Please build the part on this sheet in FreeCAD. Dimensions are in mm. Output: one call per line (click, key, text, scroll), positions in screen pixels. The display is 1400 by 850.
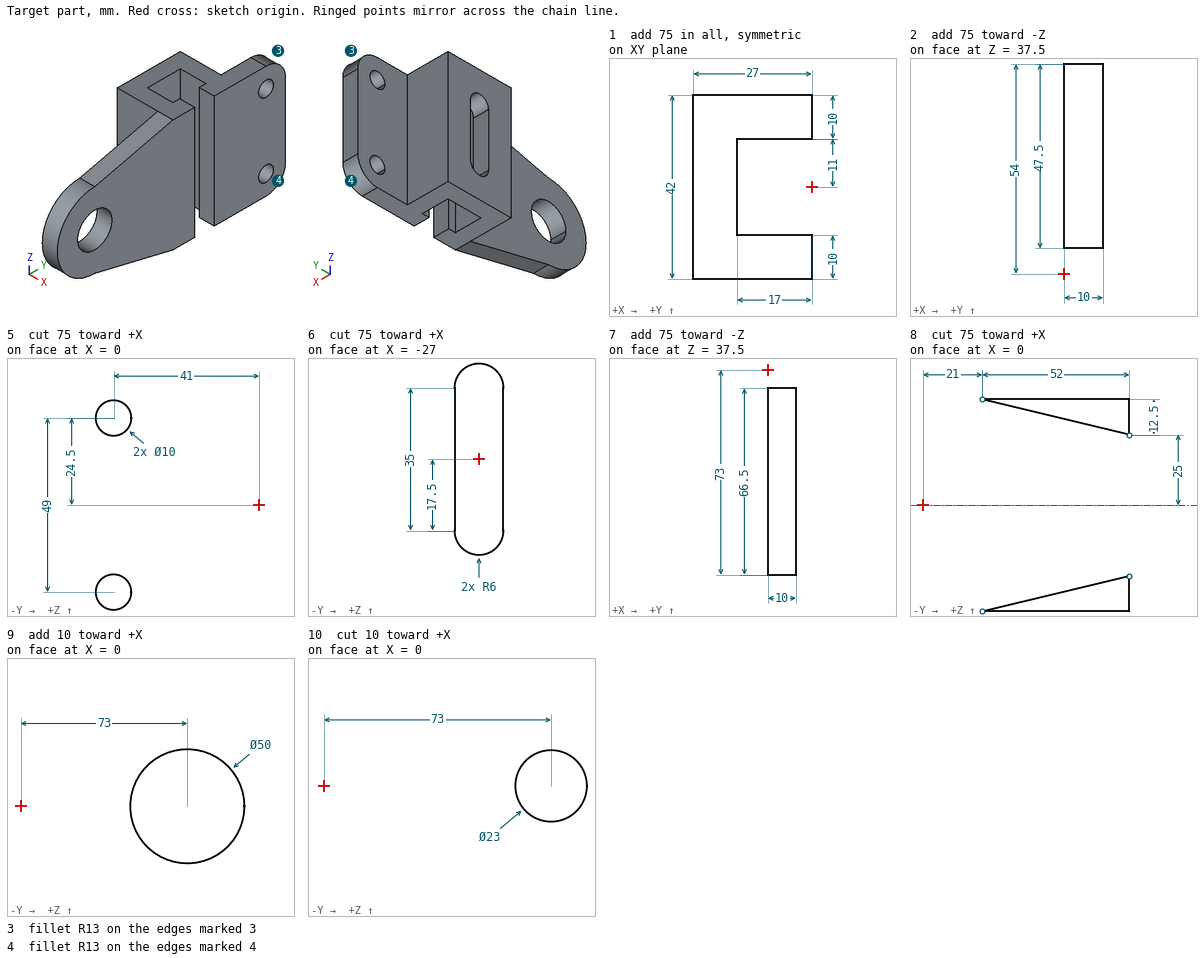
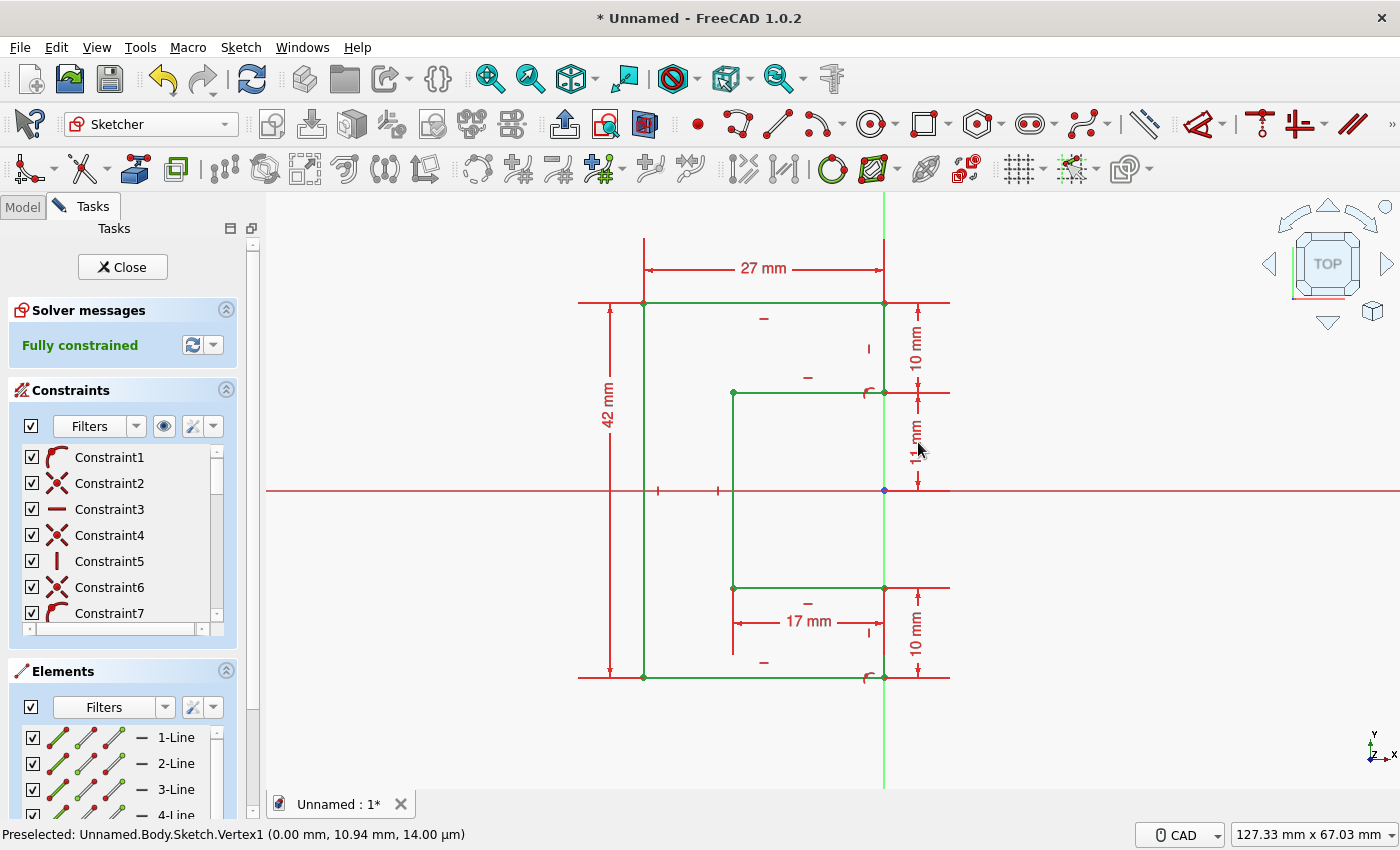
click(123, 267)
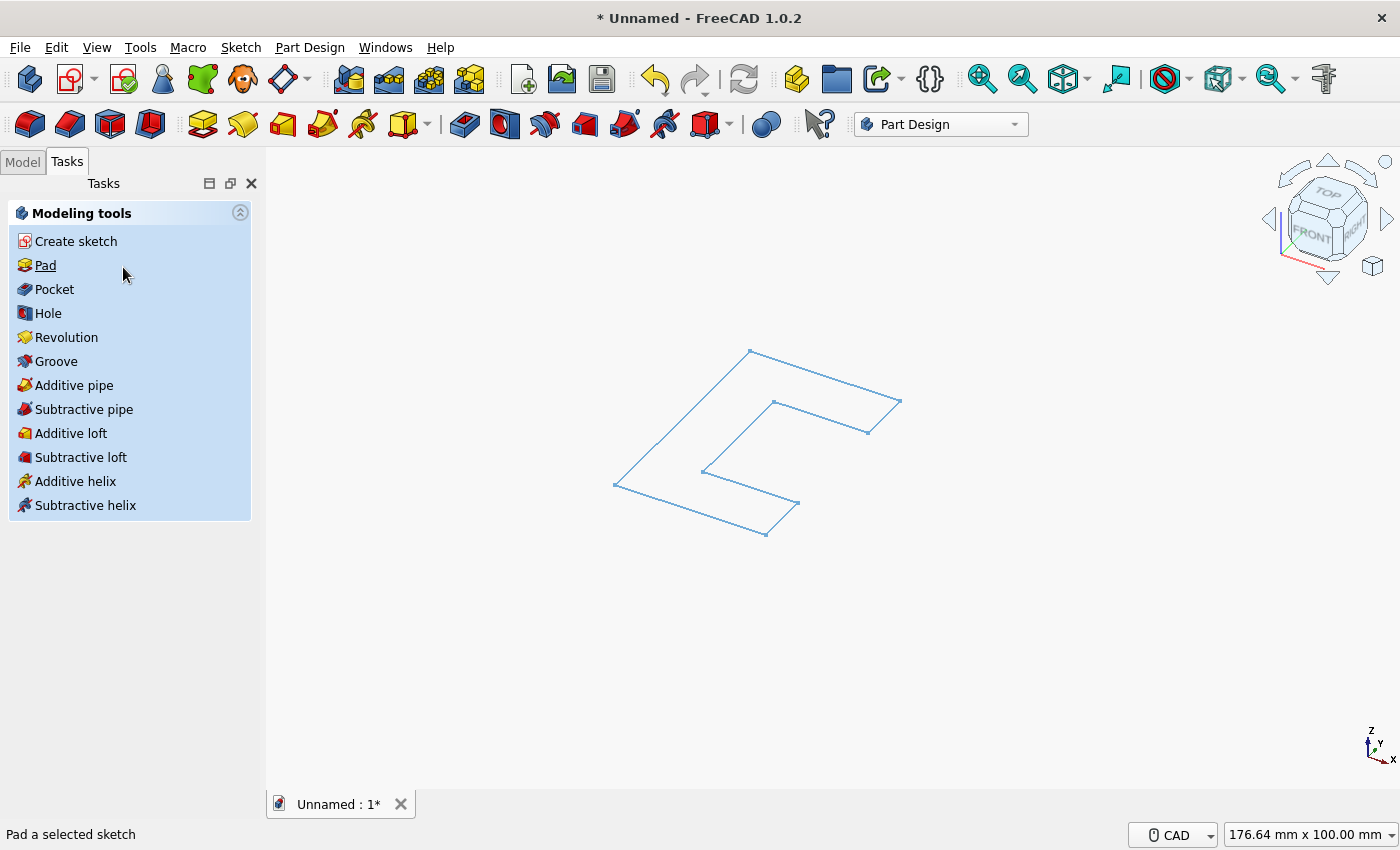
click(204, 124)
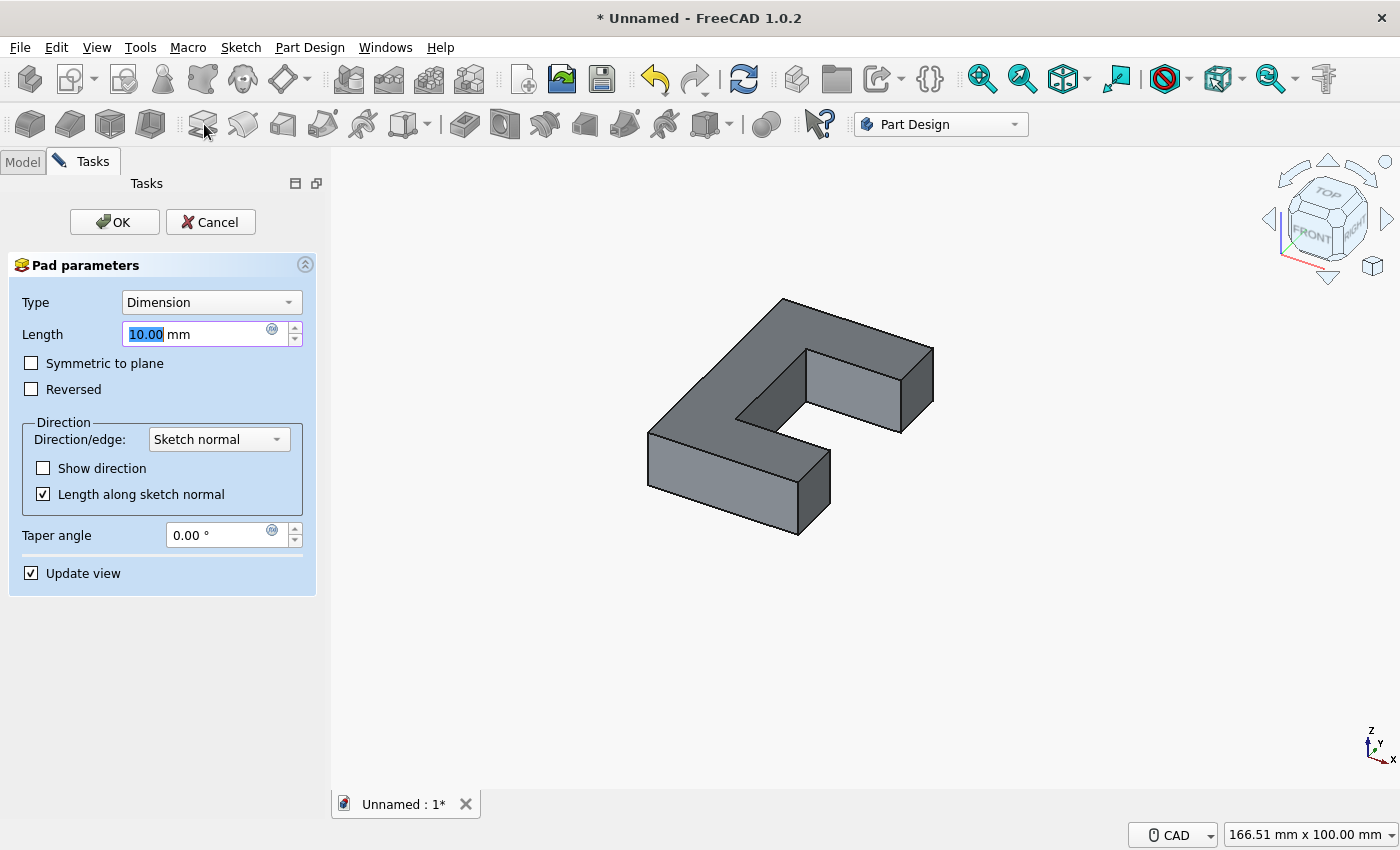
text(75)
key(Tab)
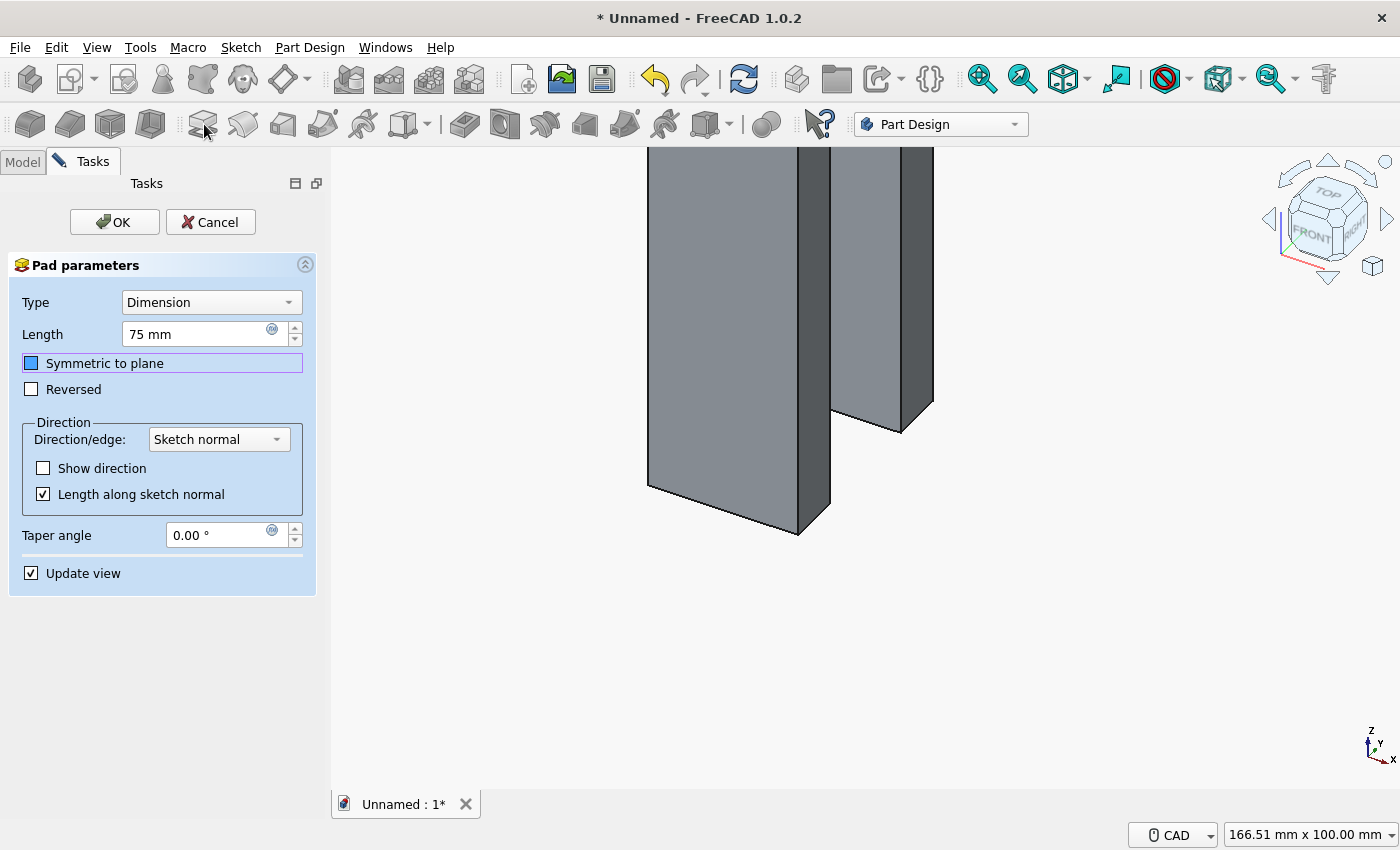
click(30, 363)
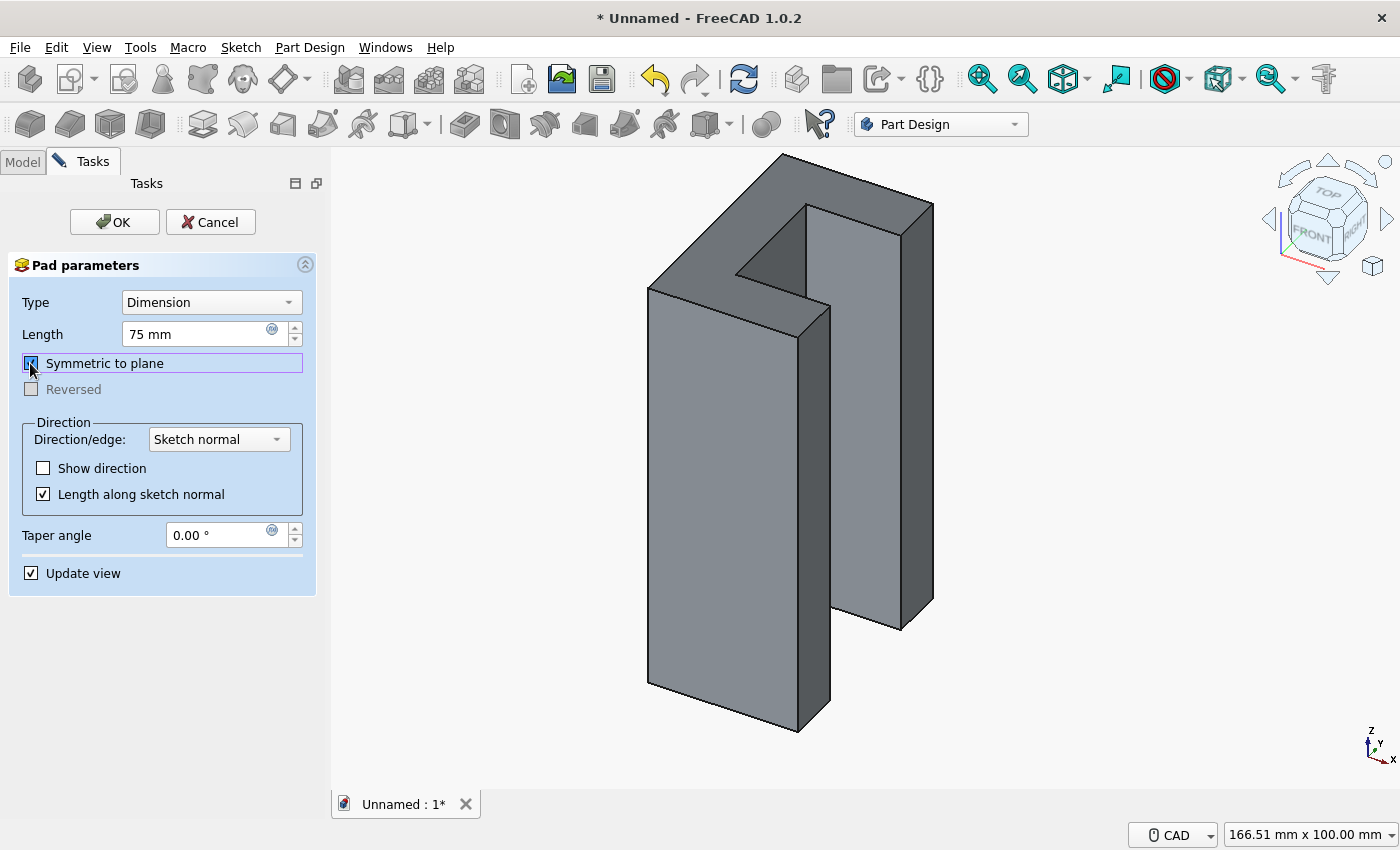
click(115, 222)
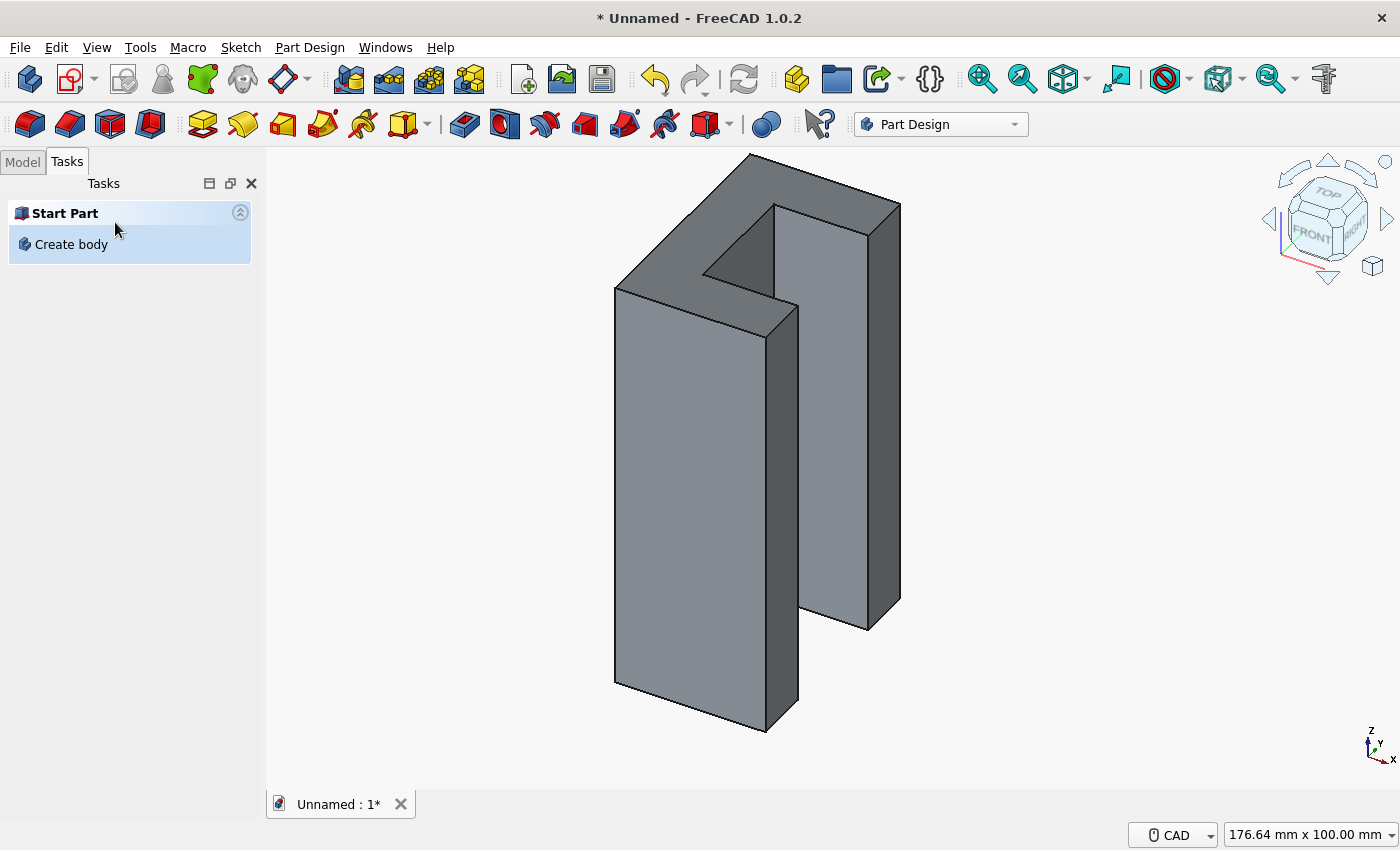
click(754, 192)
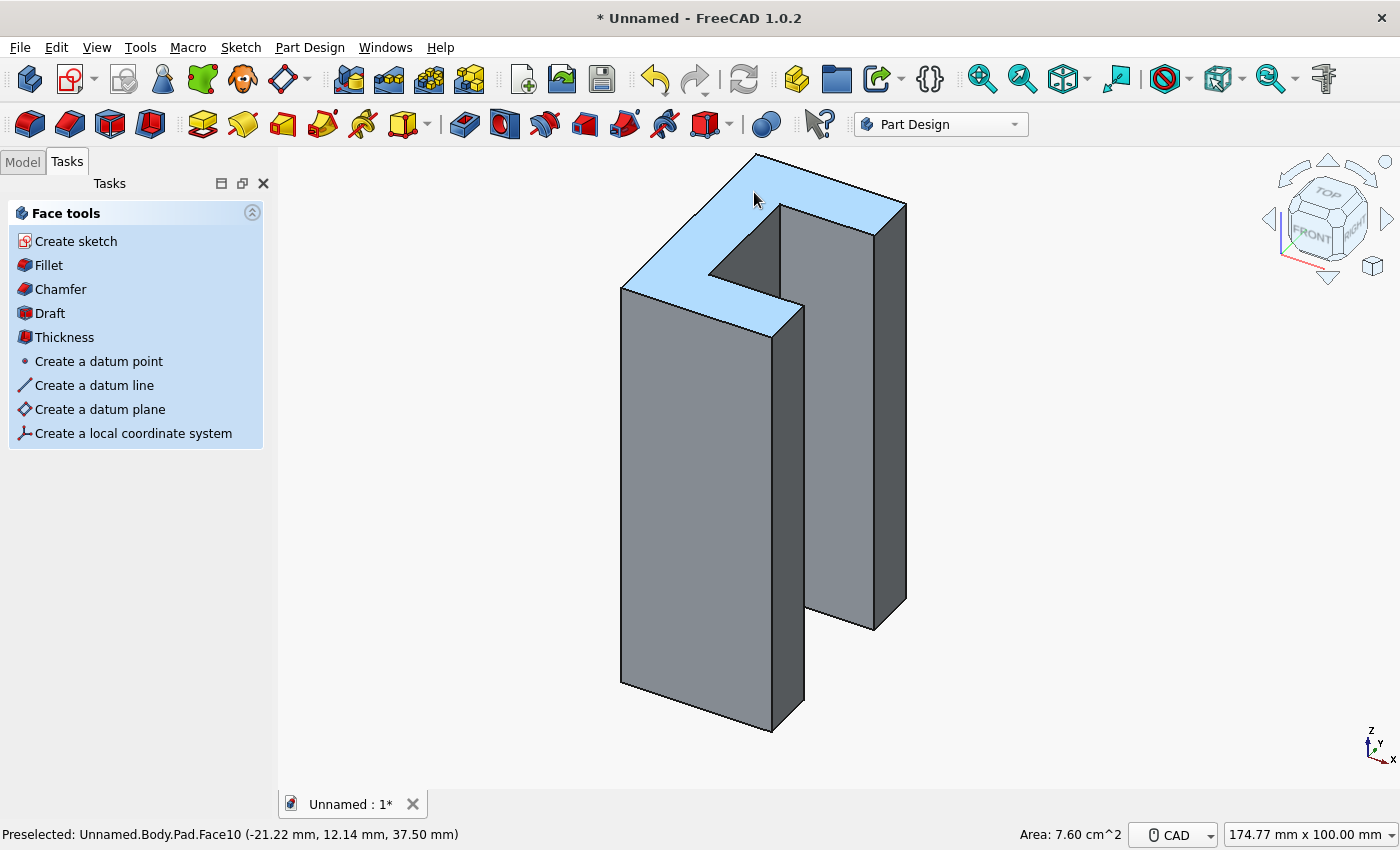
click(70, 80)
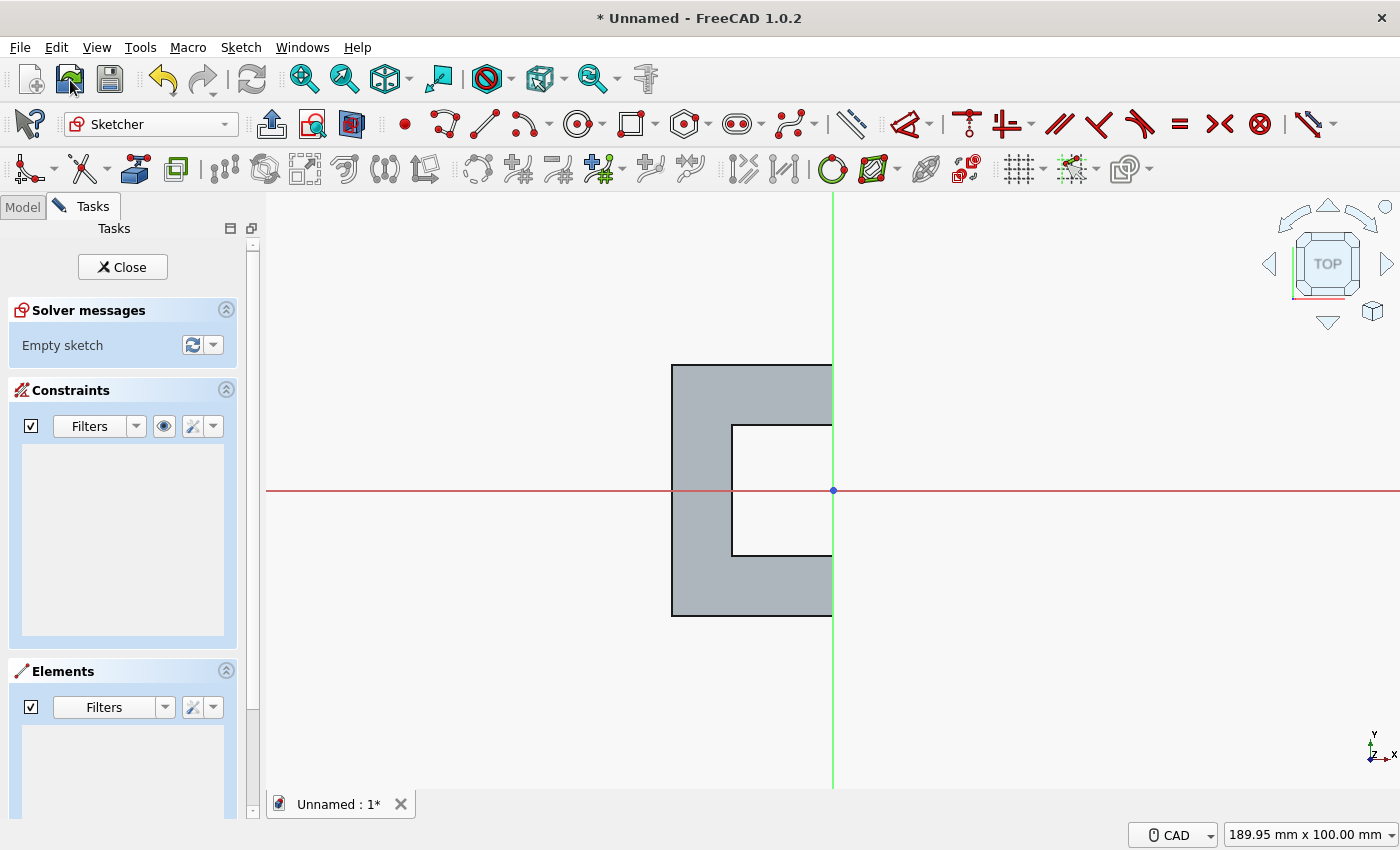
scroll(320, 761, down, 1)